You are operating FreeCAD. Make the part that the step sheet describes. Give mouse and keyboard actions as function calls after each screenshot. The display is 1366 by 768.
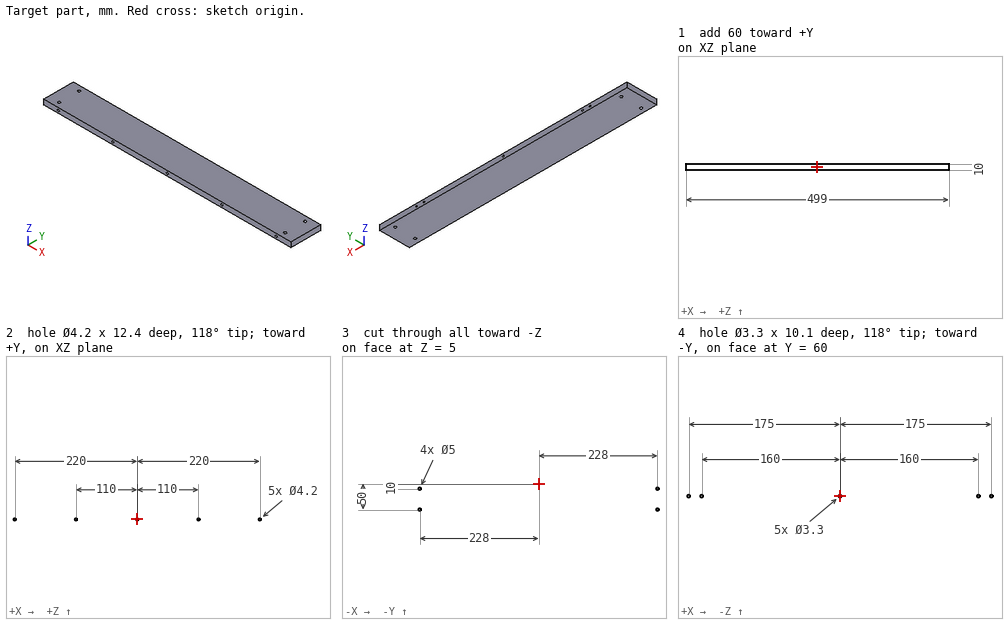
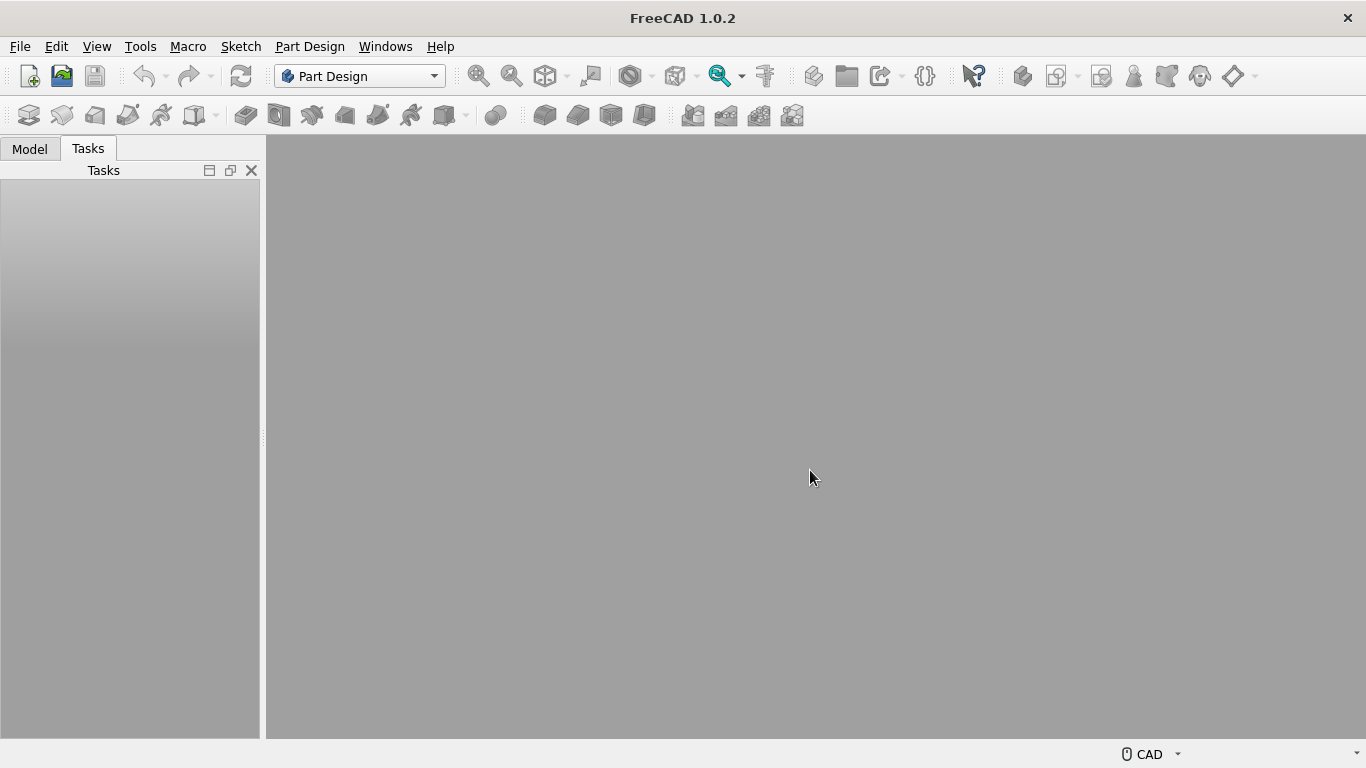
key(ctrl+n)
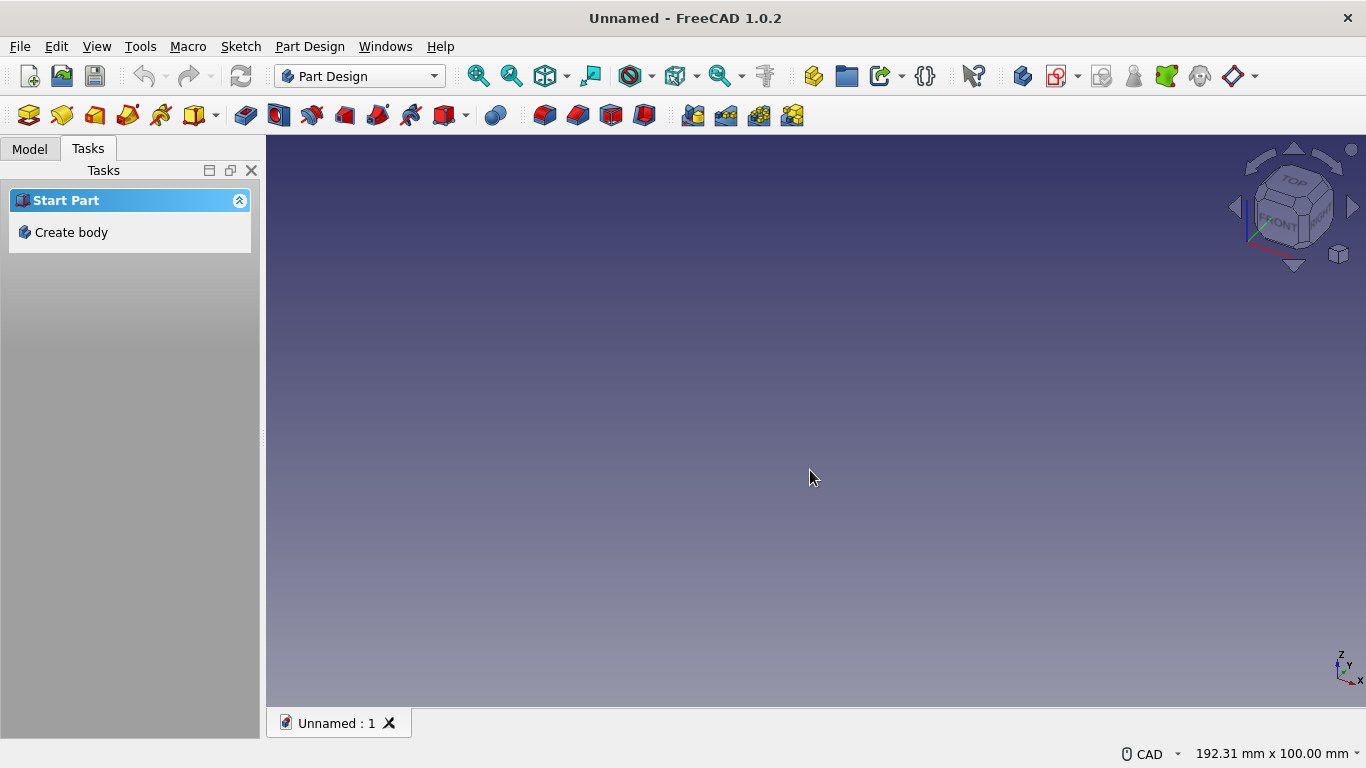
click(1056, 76)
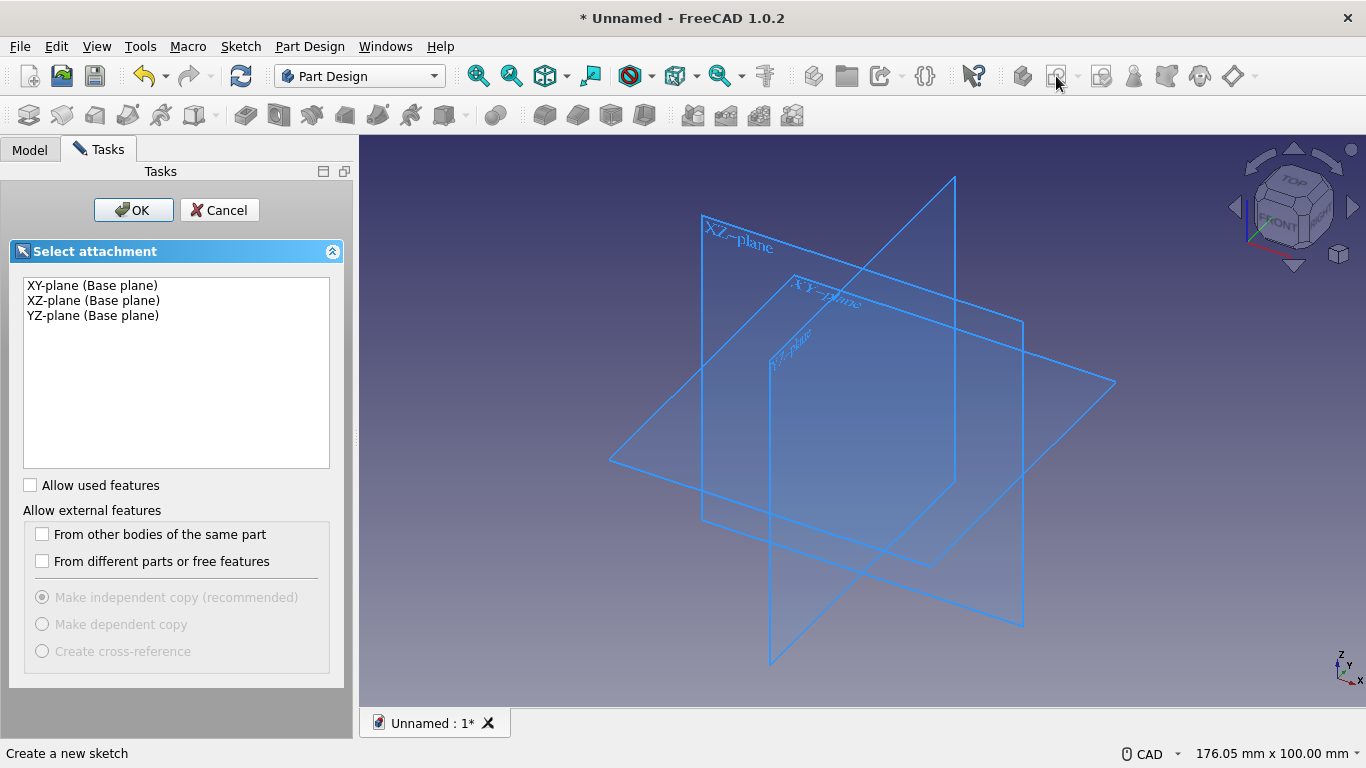
click(84, 300)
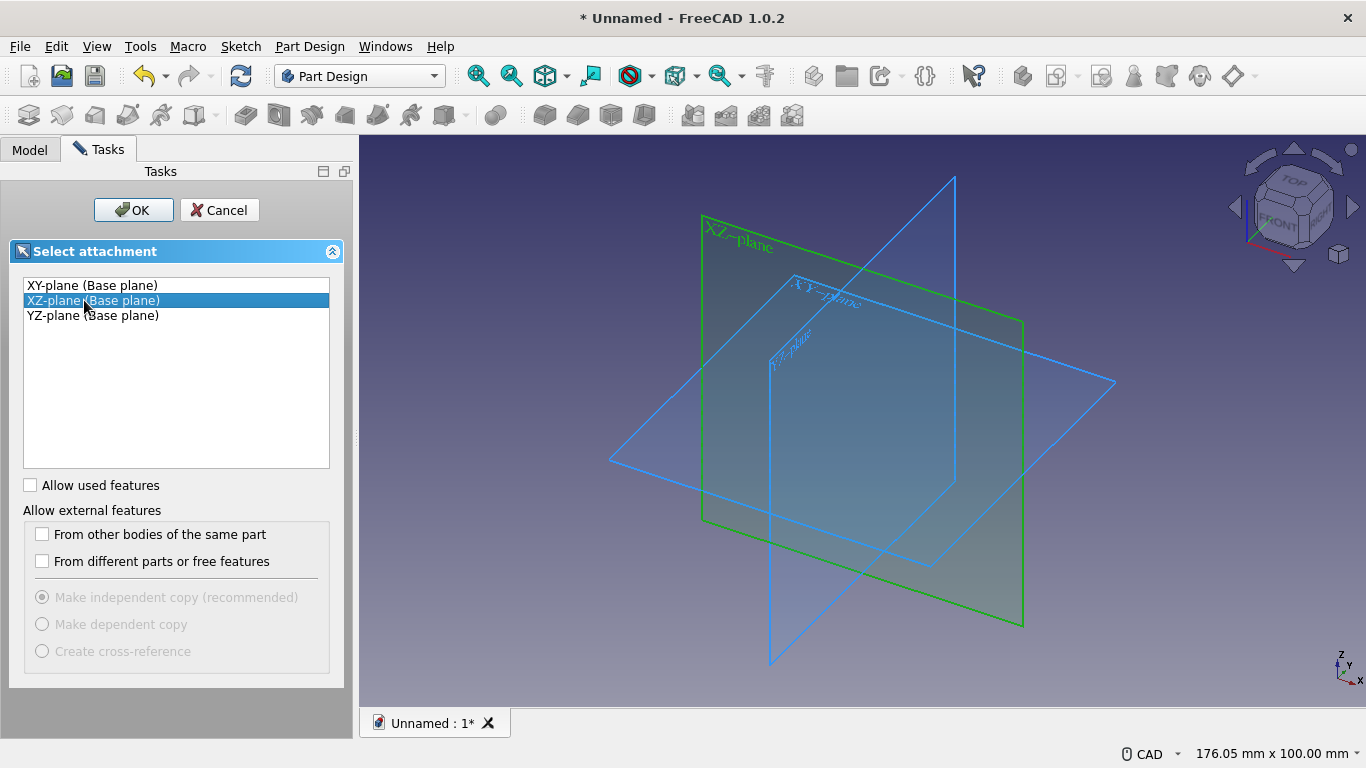
click(134, 210)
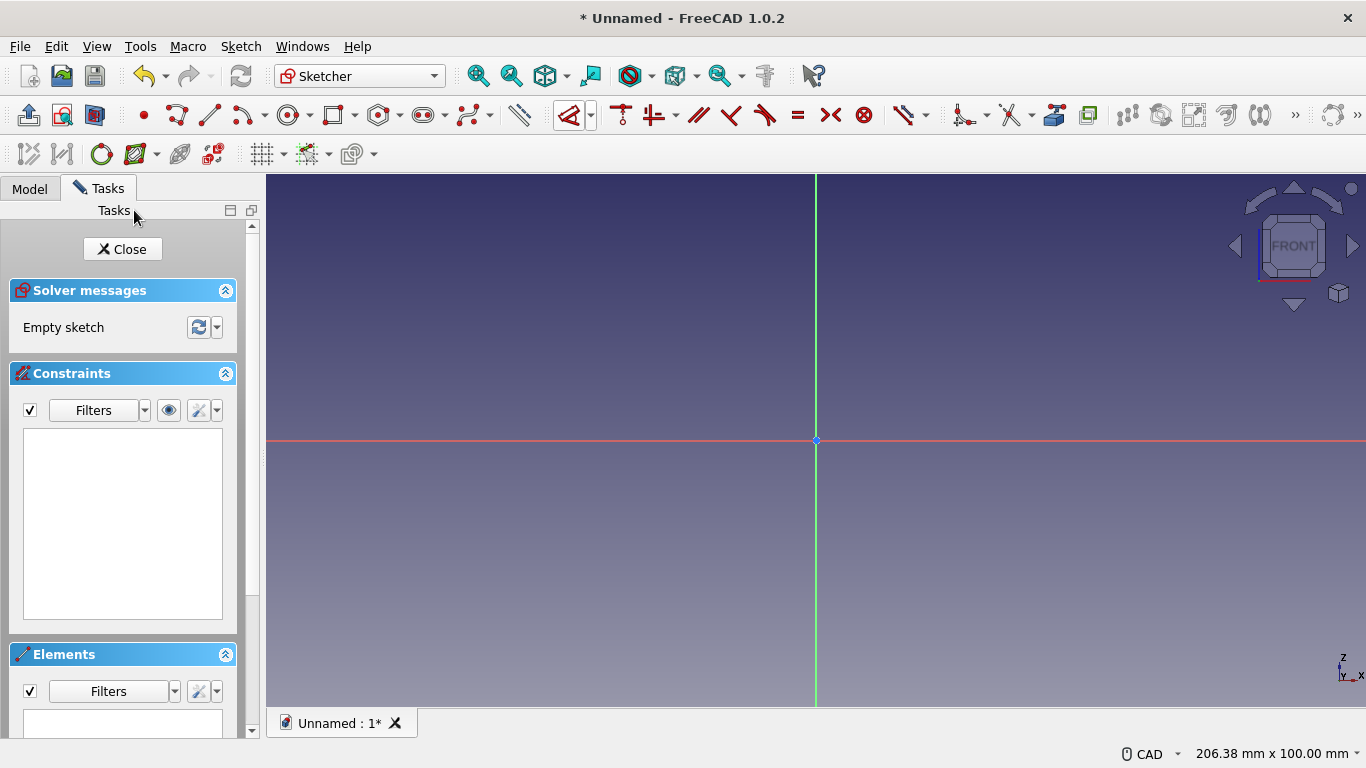
scroll(725, 440, down, 7)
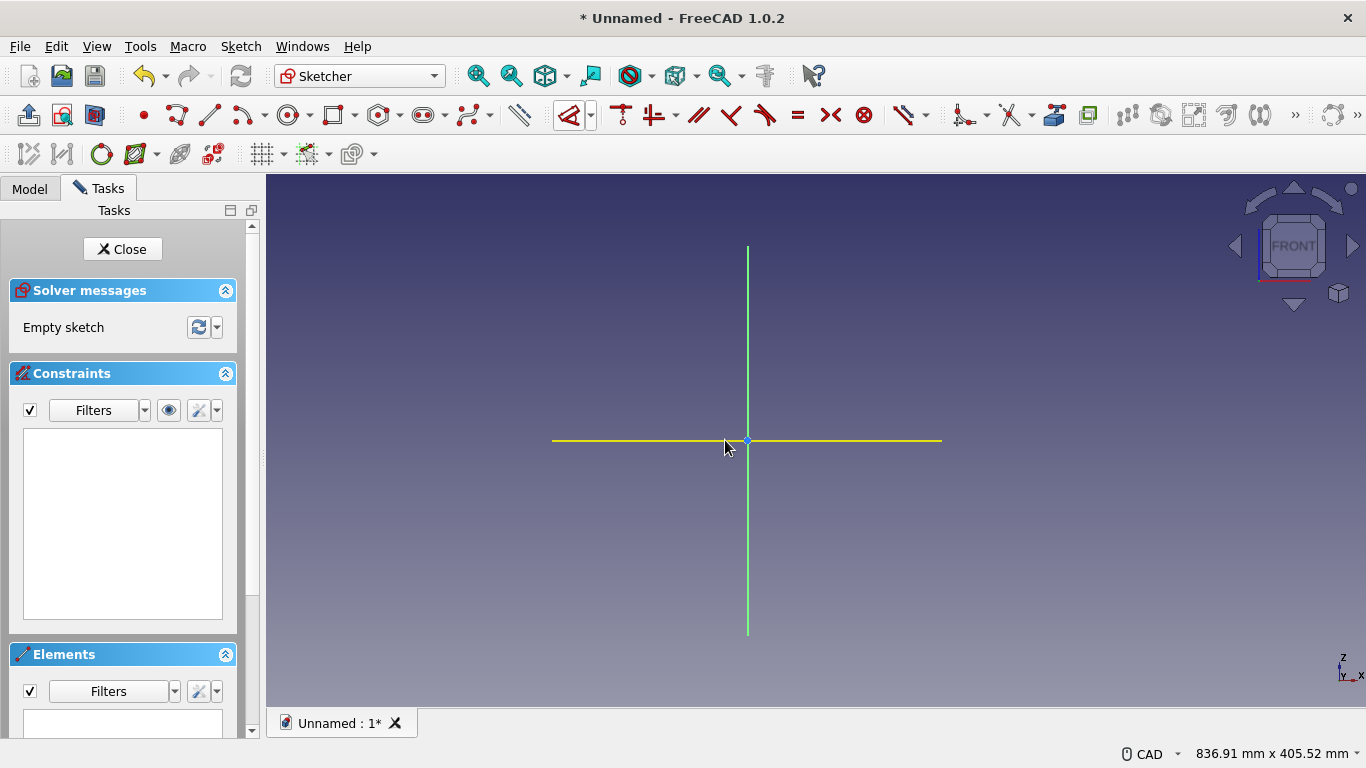
click(354, 116)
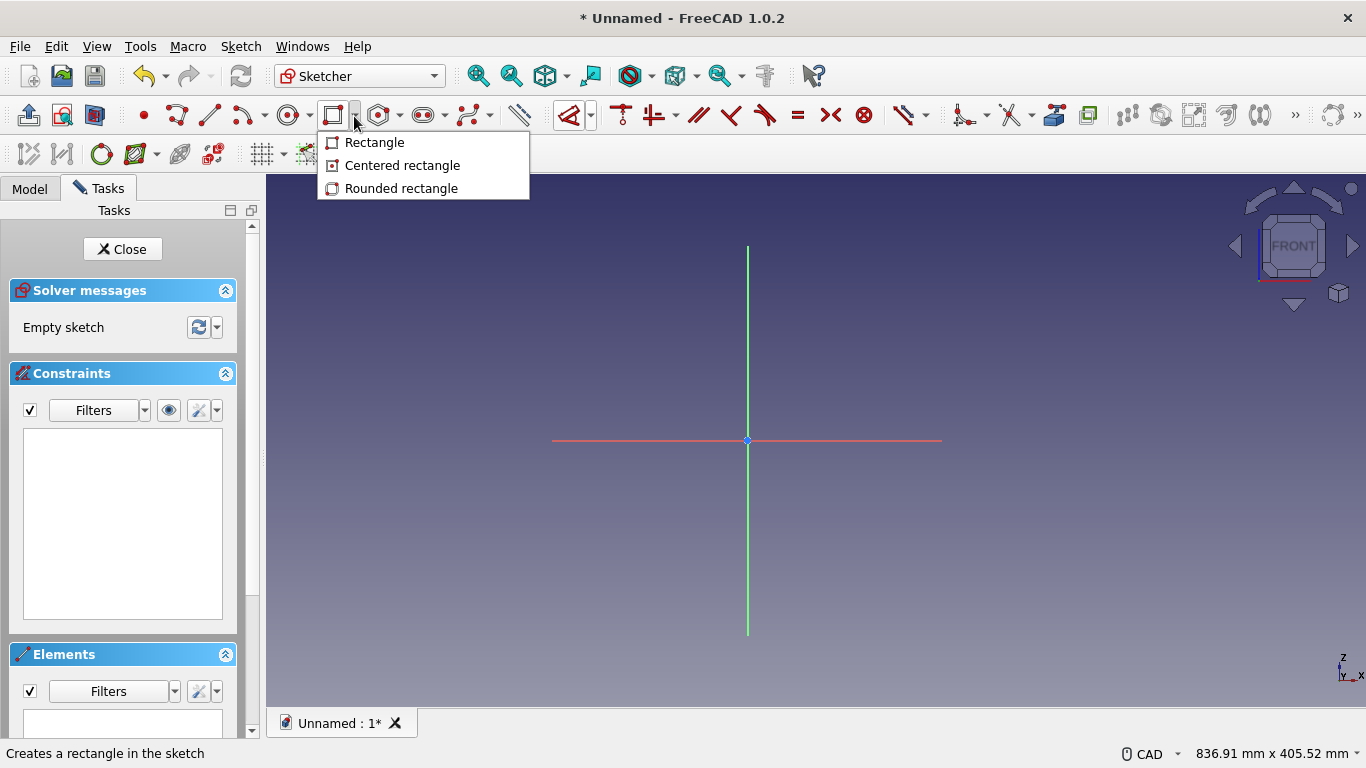
click(424, 166)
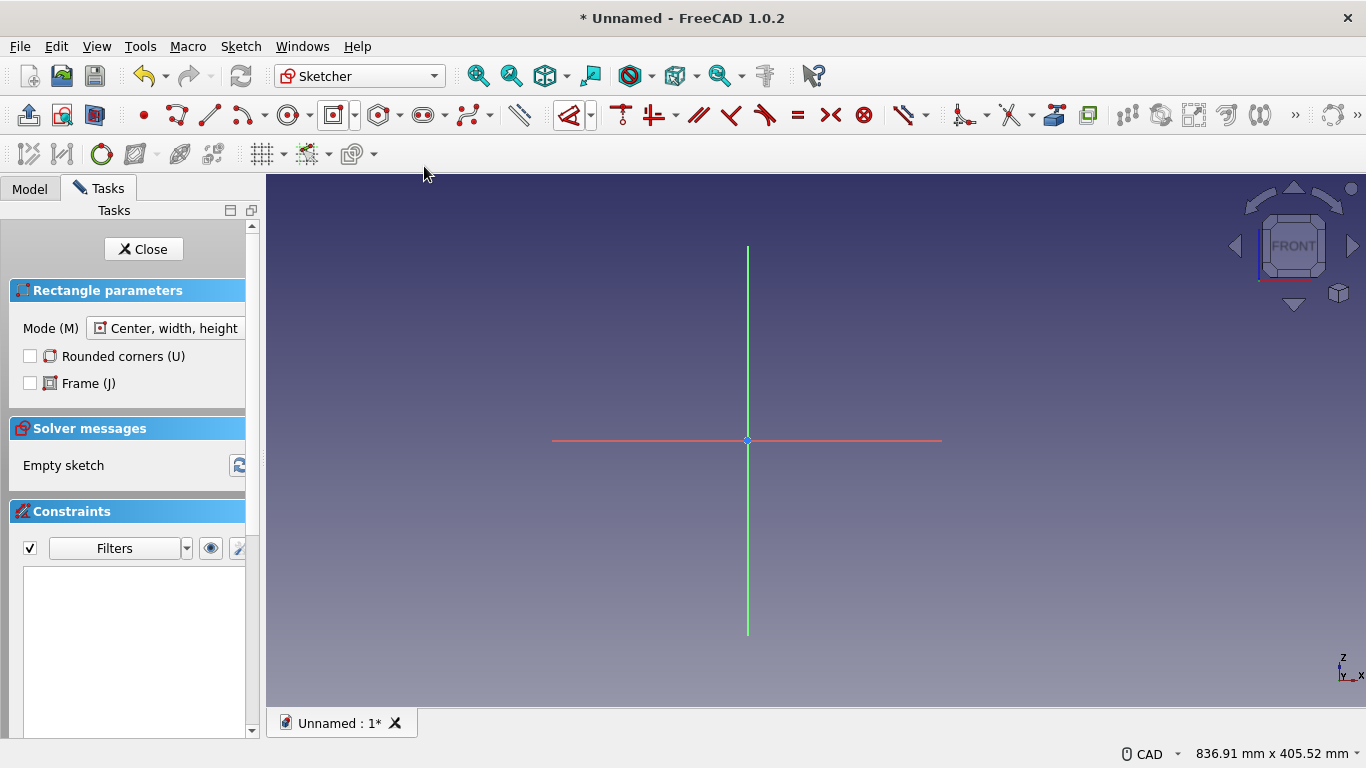
scroll(748, 440, up, 5)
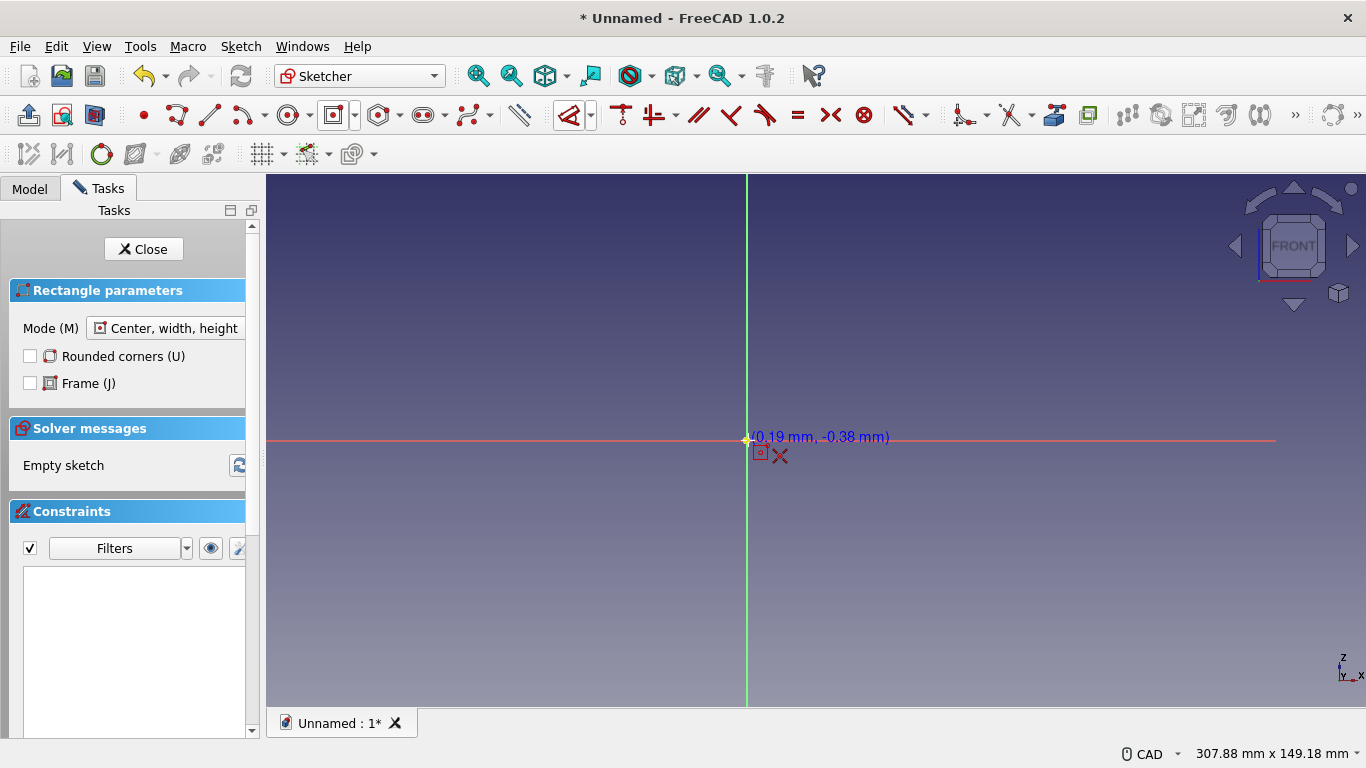
click(747, 440)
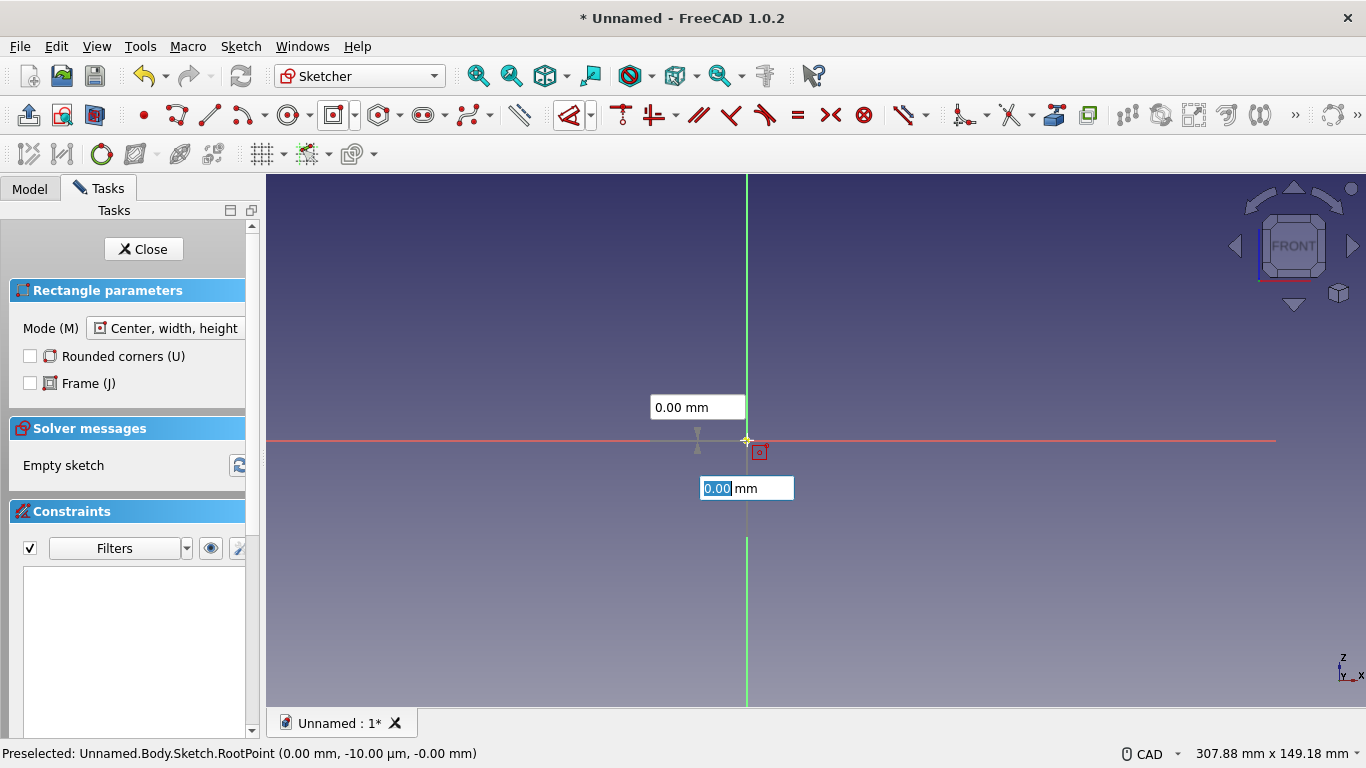
scroll(748, 440, down, 5)